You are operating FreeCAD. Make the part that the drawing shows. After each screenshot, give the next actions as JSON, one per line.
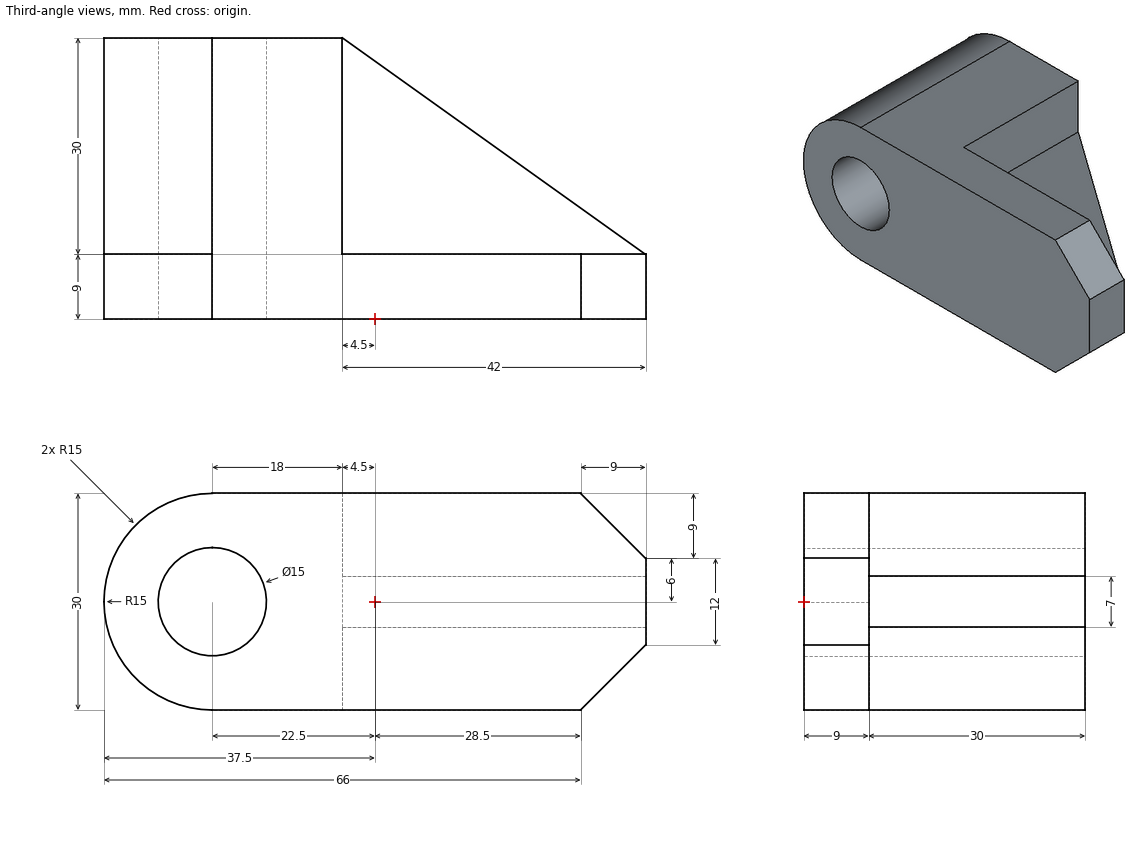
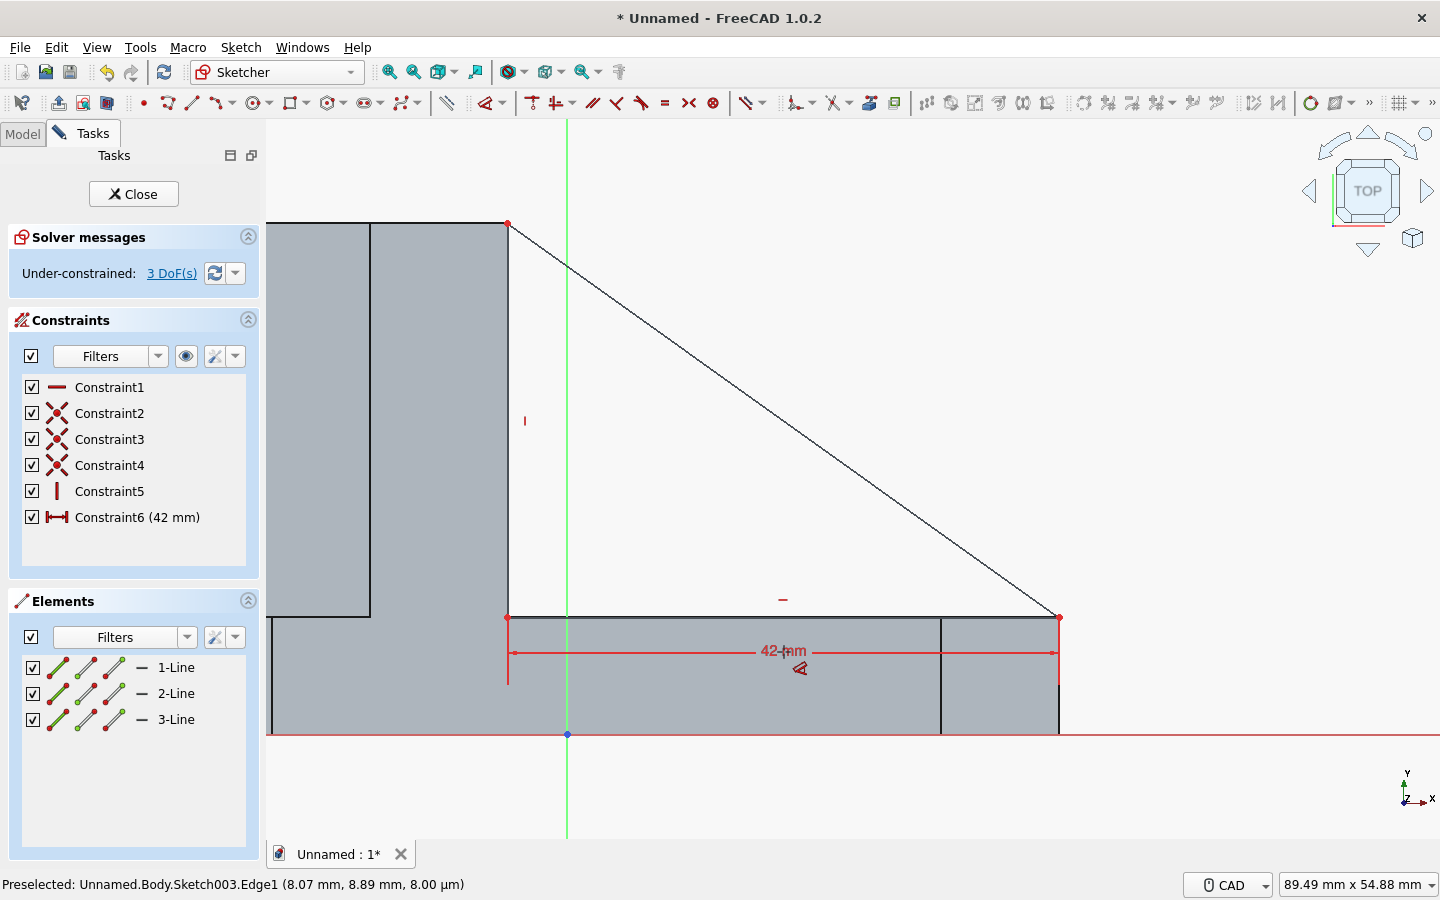
{"action": "left_click", "coordinate": [508, 342]}
{"action": "left_click", "coordinate": [474, 421]}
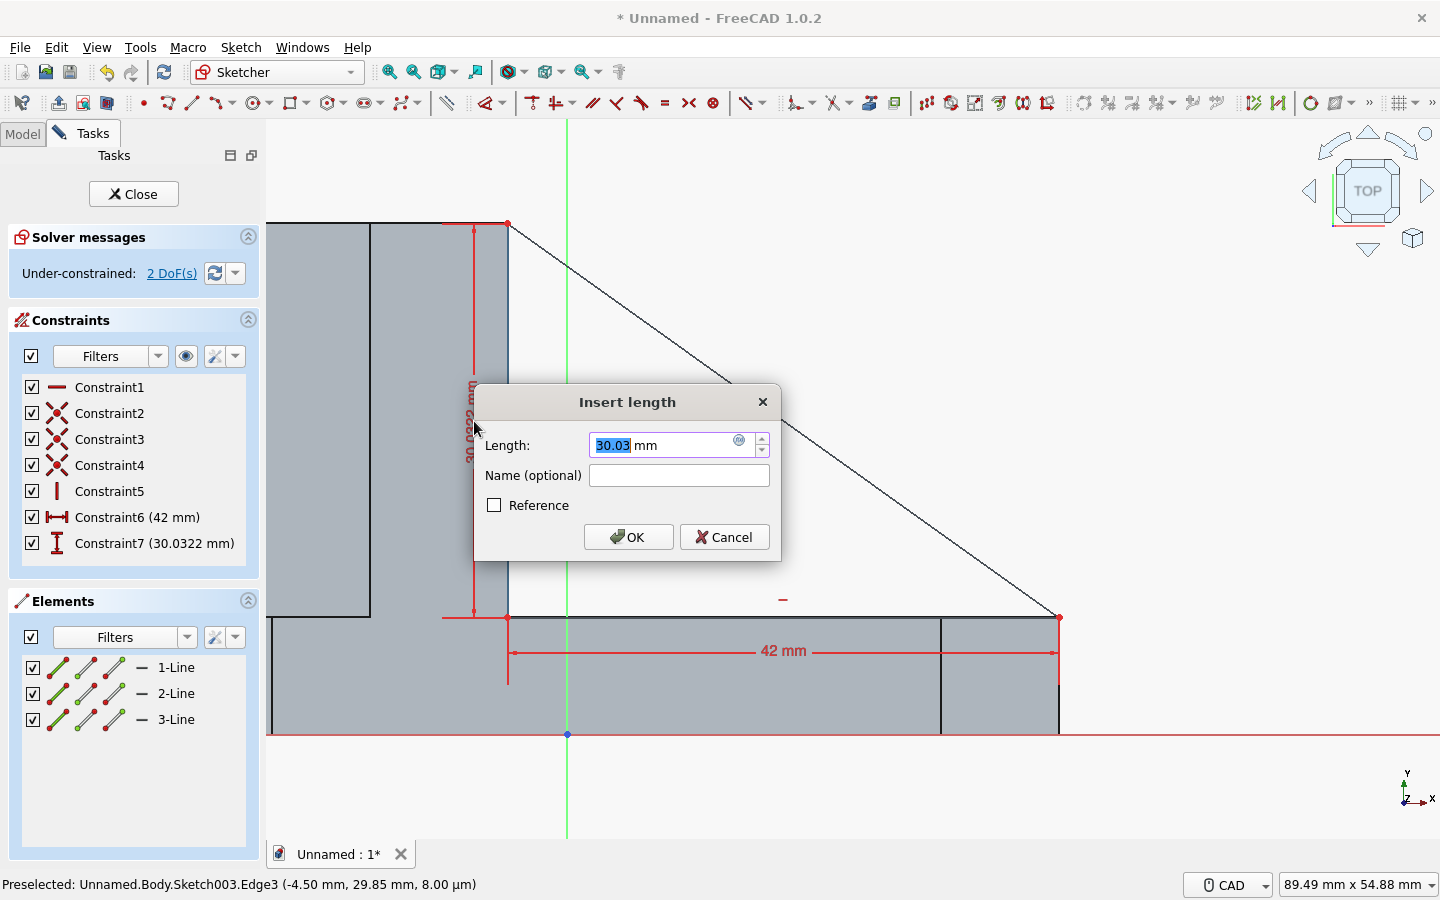
{"action": "type", "text": "30"}
{"action": "key", "text": "Return"}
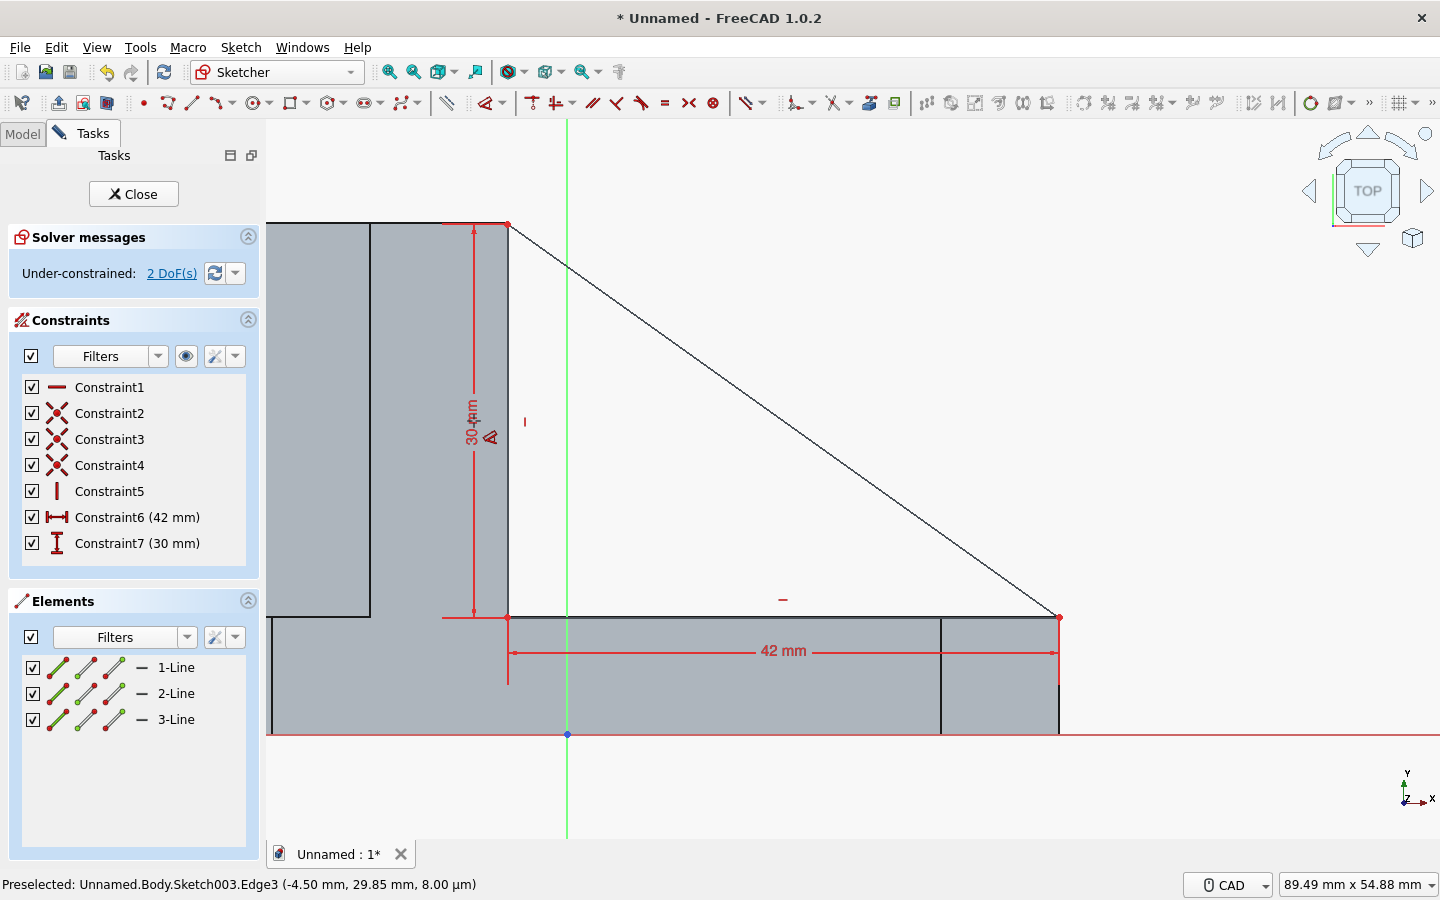
{"action": "left_click", "coordinate": [508, 618]}
{"action": "left_click", "coordinate": [474, 676]}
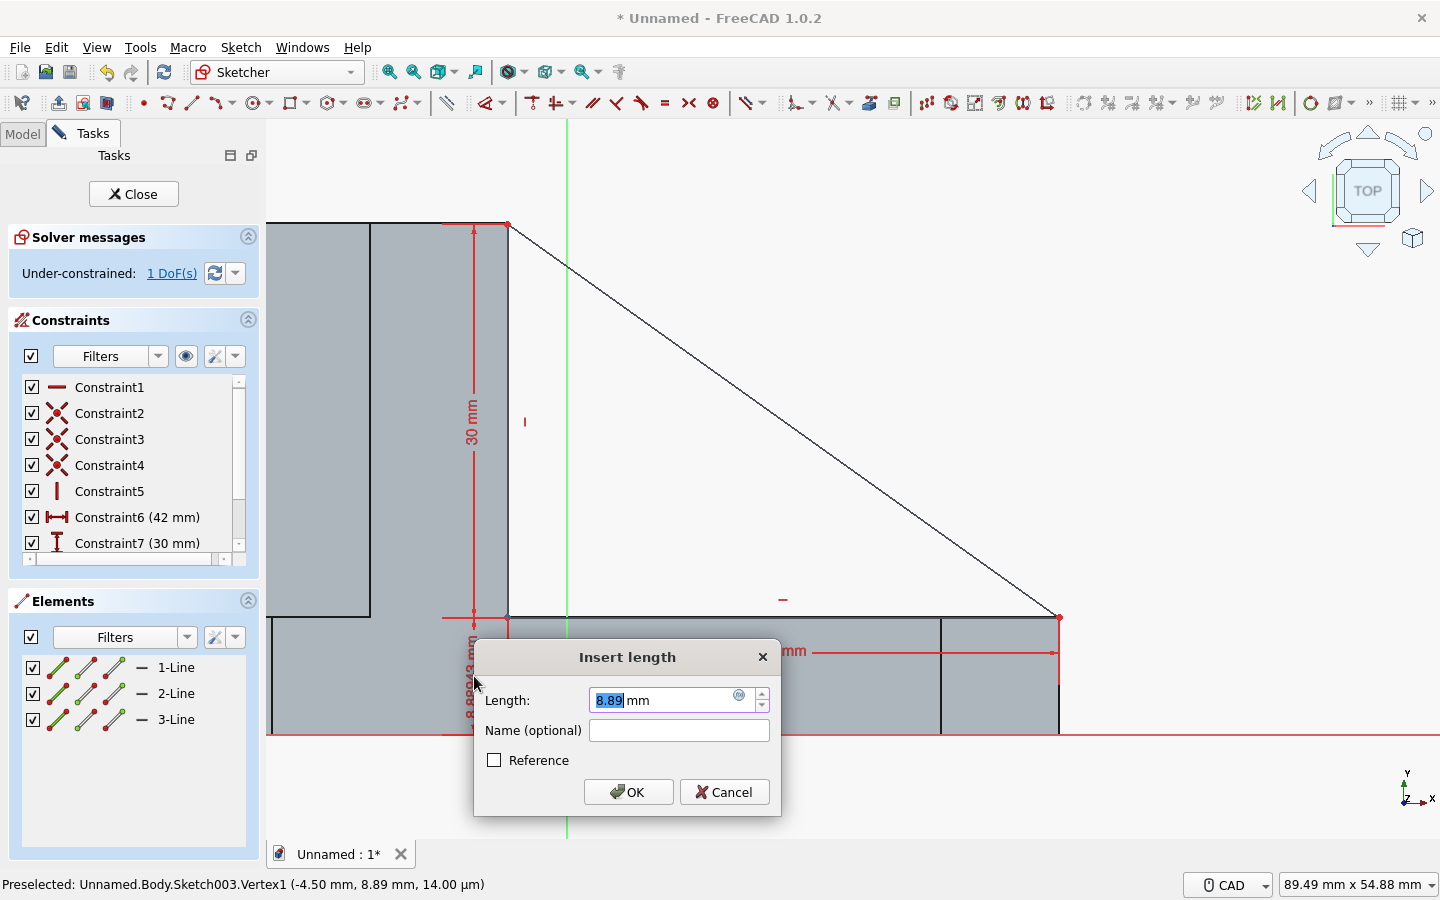
{"action": "type", "text": "9"}
{"action": "key", "text": "Return"}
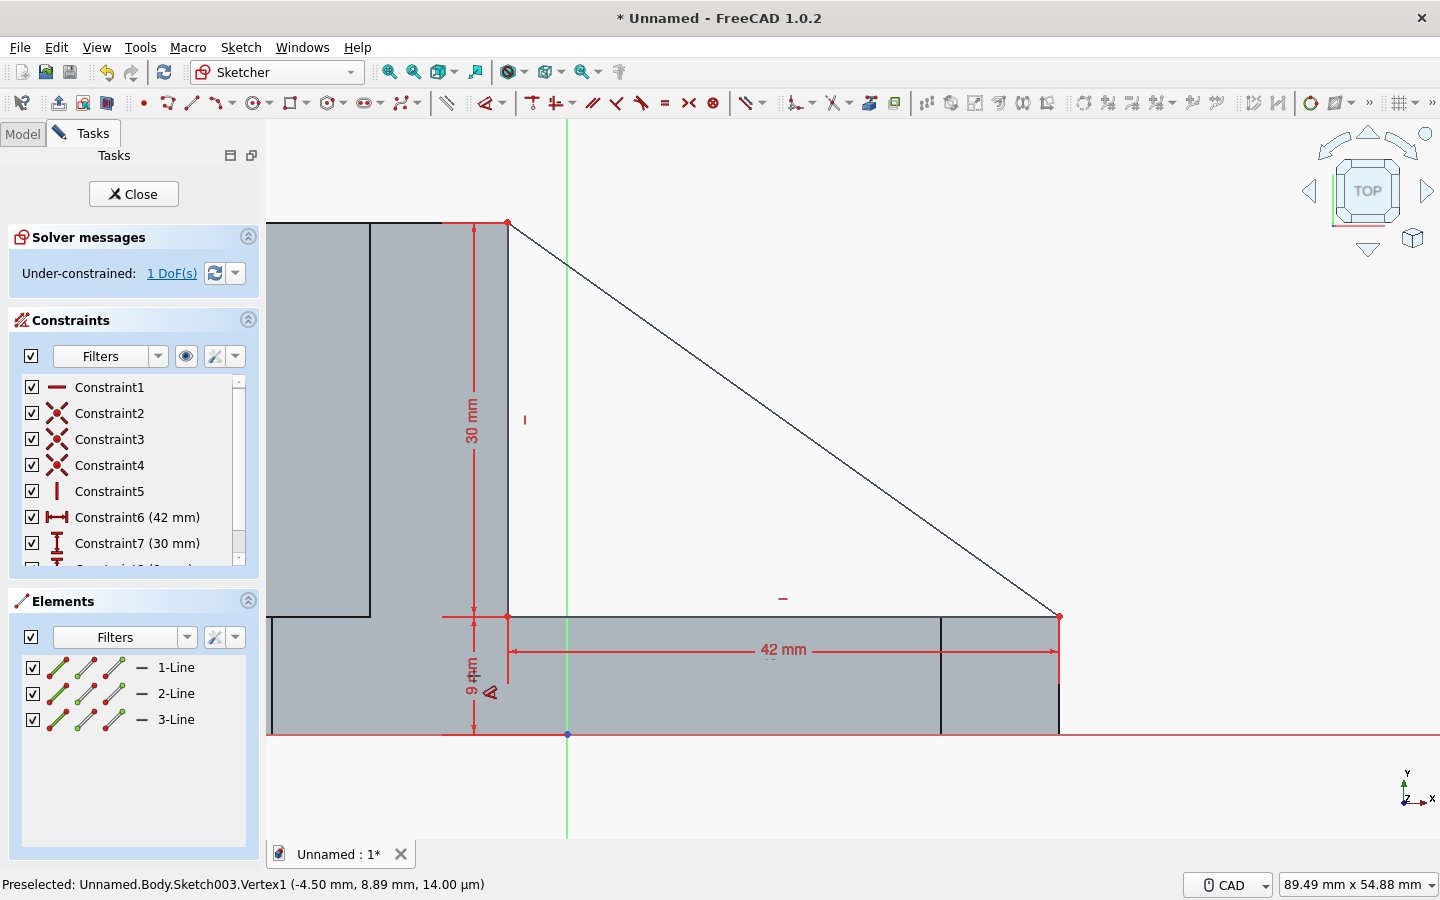
{"action": "left_click", "coordinate": [508, 617]}
{"action": "left_click", "coordinate": [538, 769]}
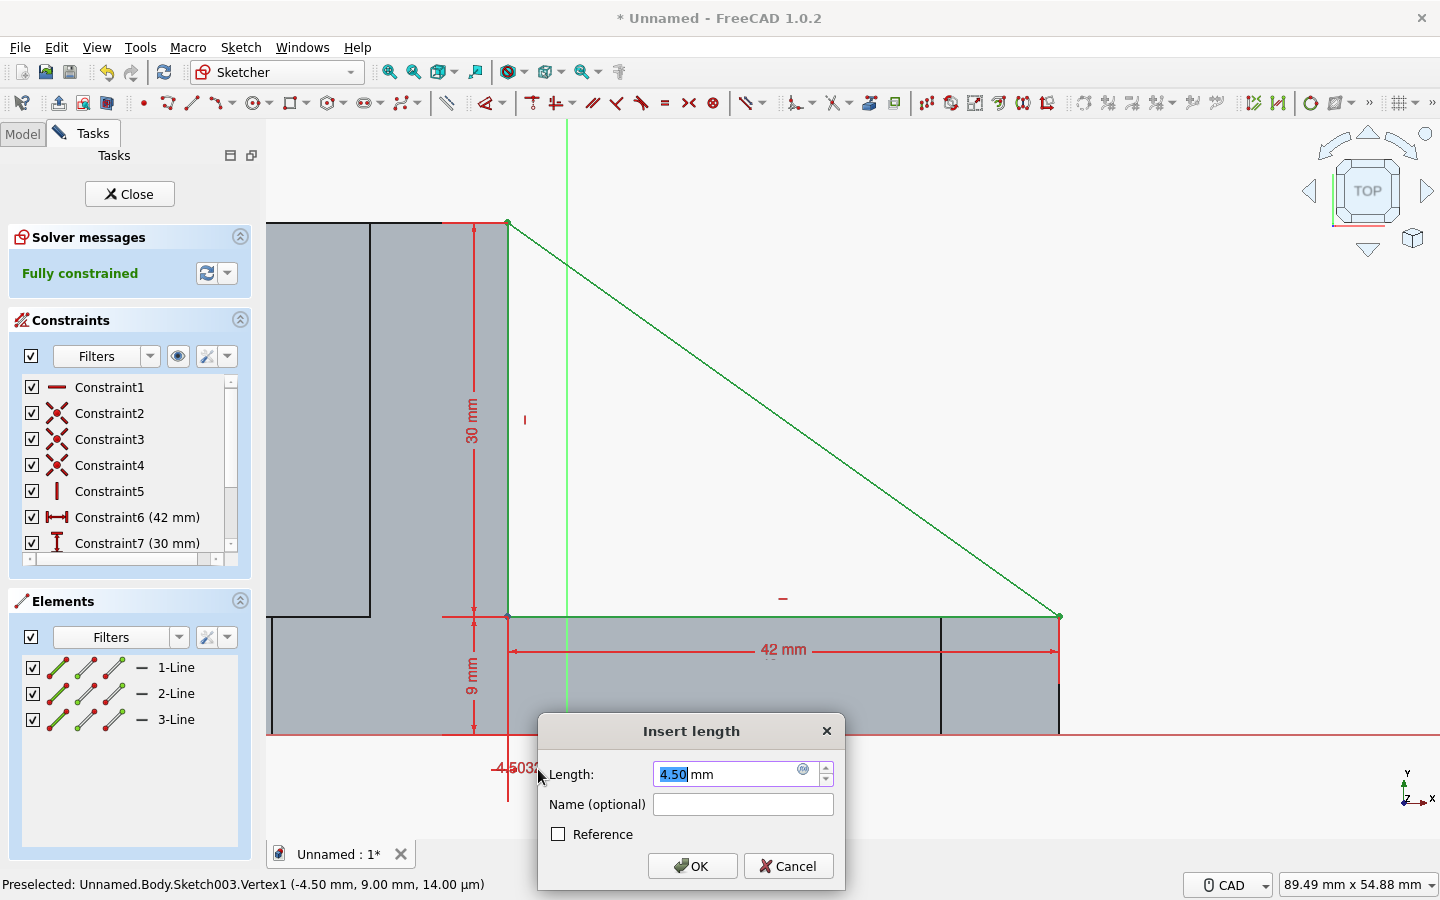
{"action": "type", "text": "4.5"}
{"action": "key", "text": "Return"}
{"action": "key", "text": "Escape"}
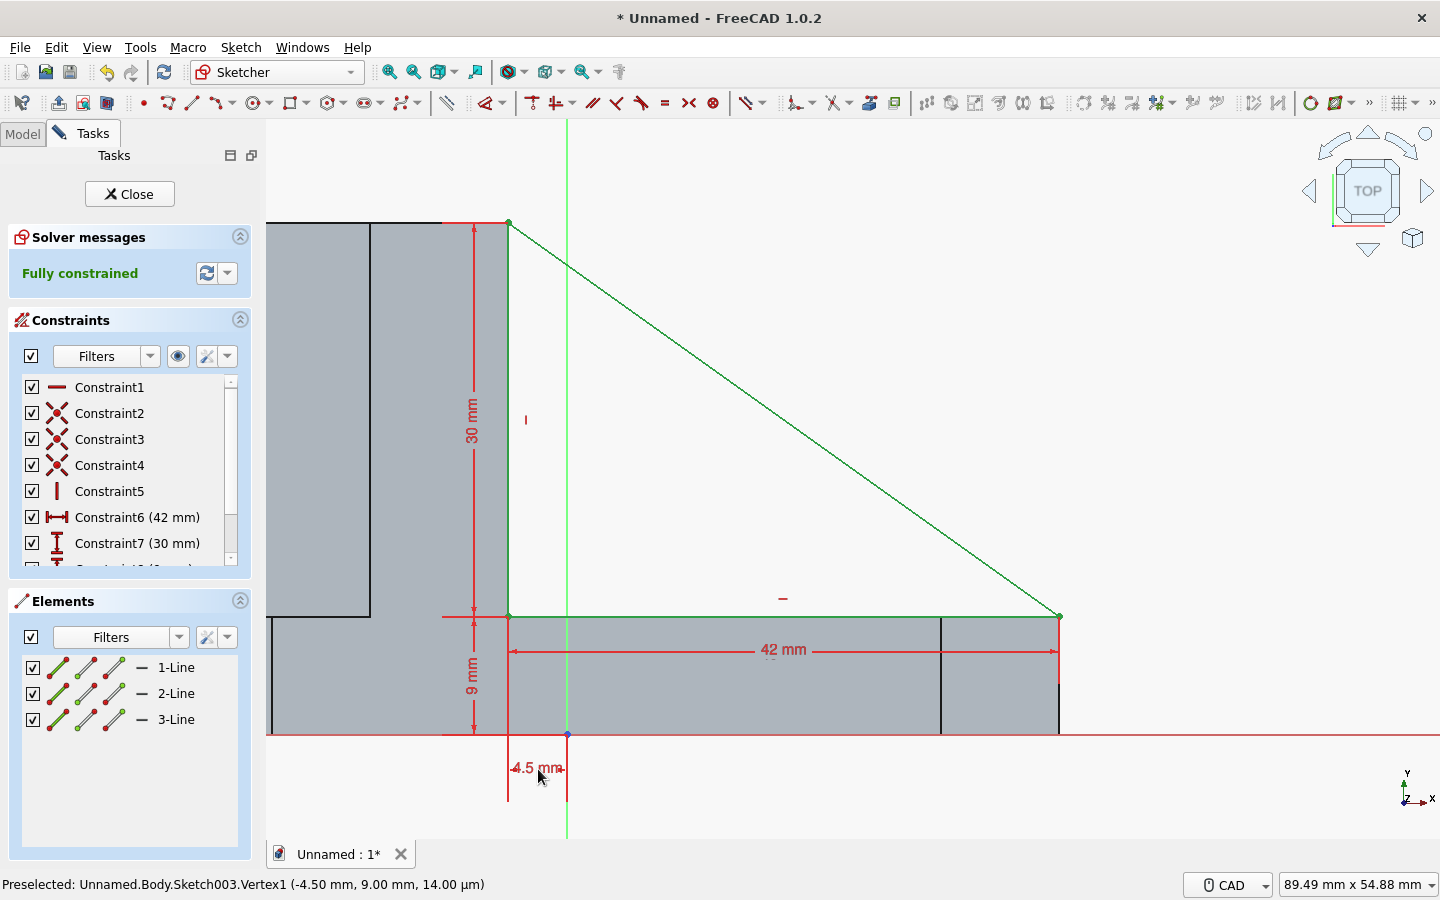
{"action": "left_click", "coordinate": [130, 194]}